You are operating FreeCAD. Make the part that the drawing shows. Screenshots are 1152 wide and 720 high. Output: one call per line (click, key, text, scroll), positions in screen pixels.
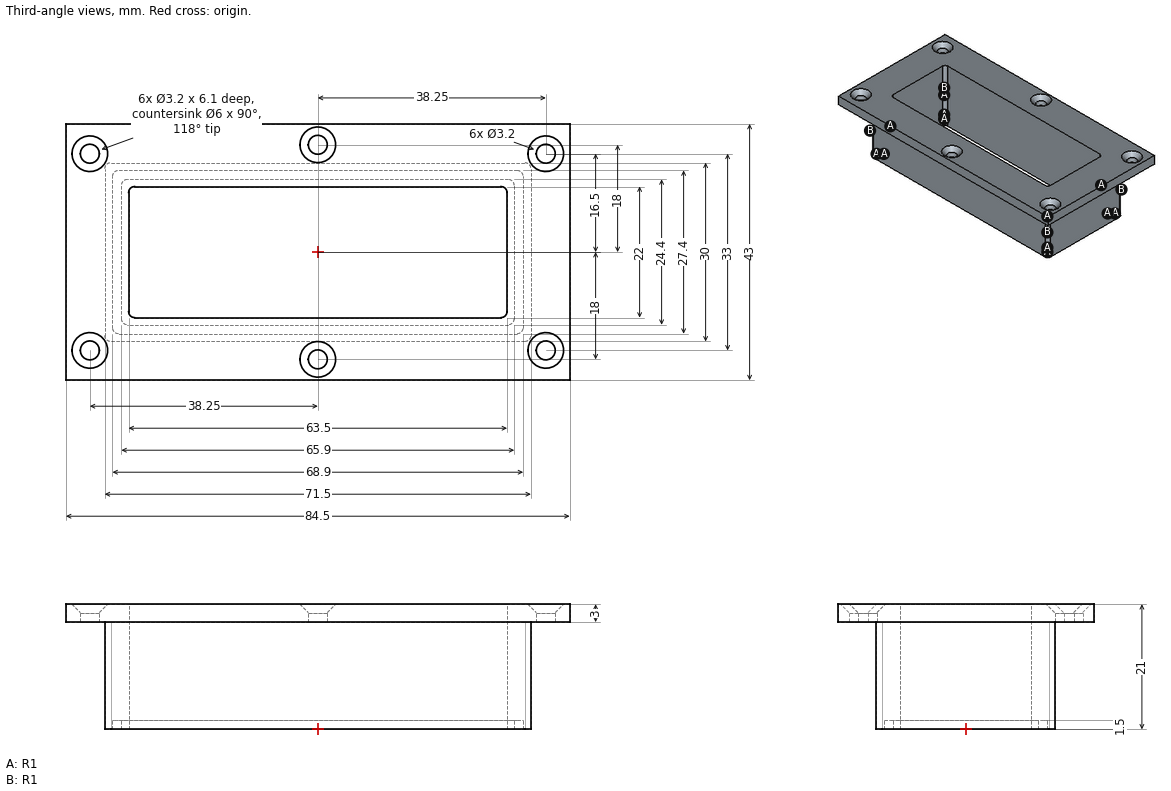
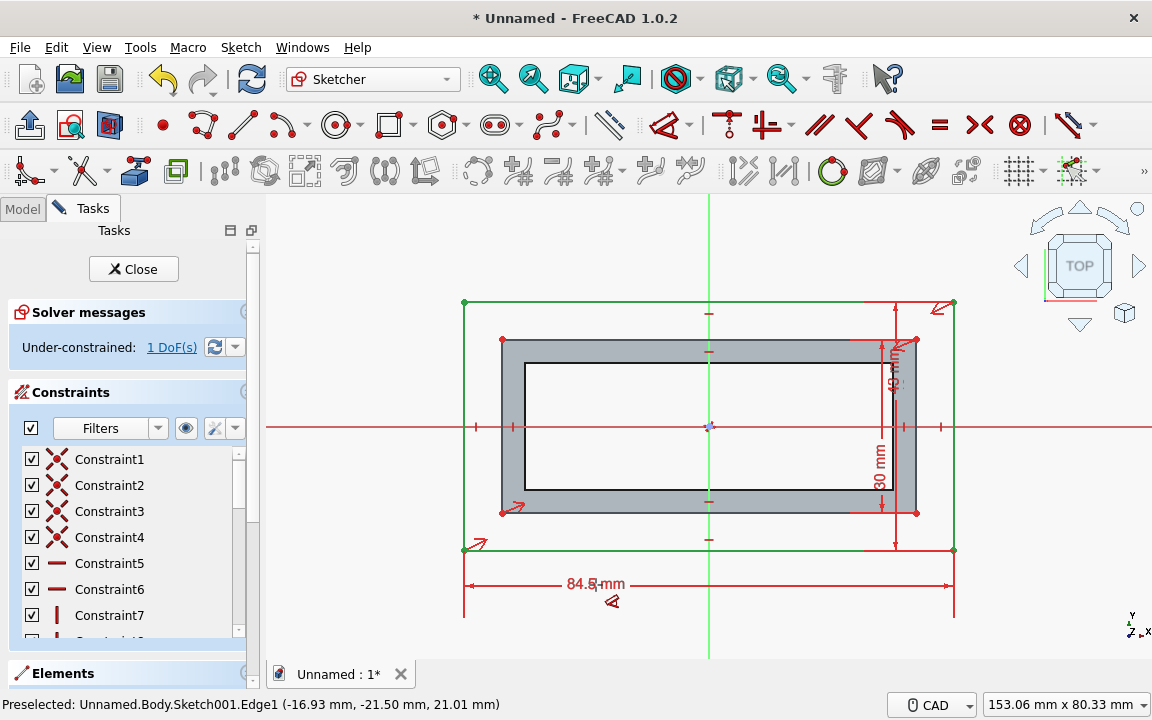
click(626, 513)
click(614, 479)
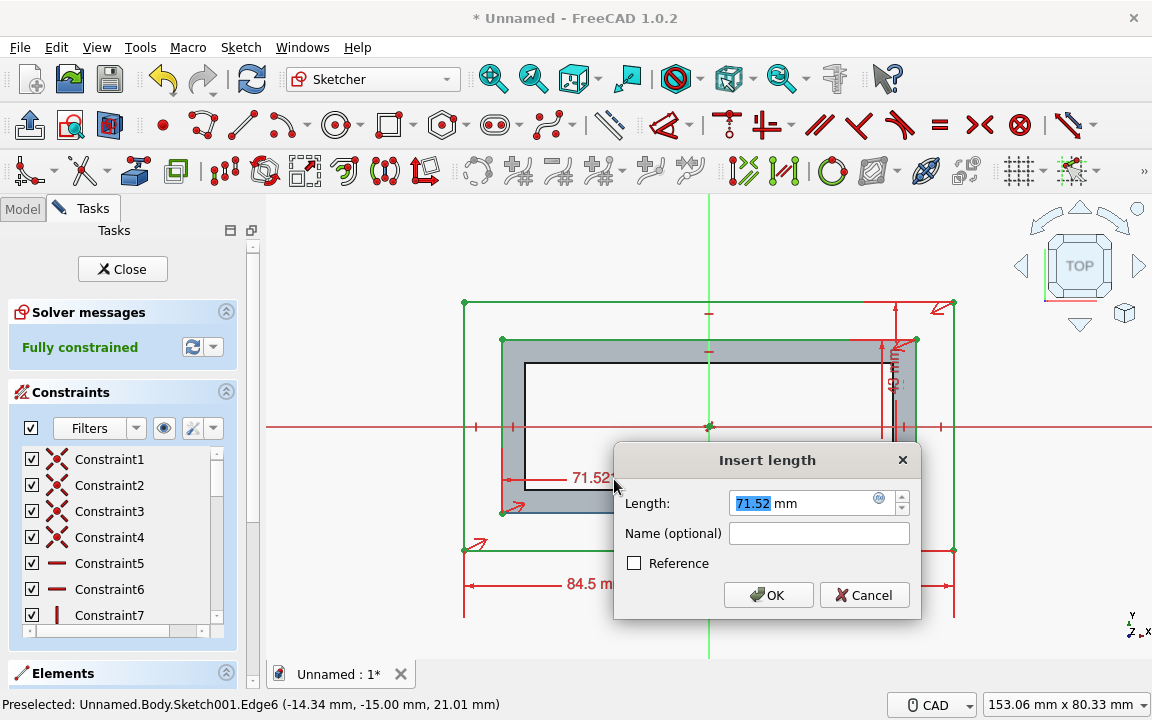
text(71.5)
key(Return)
key(Escape)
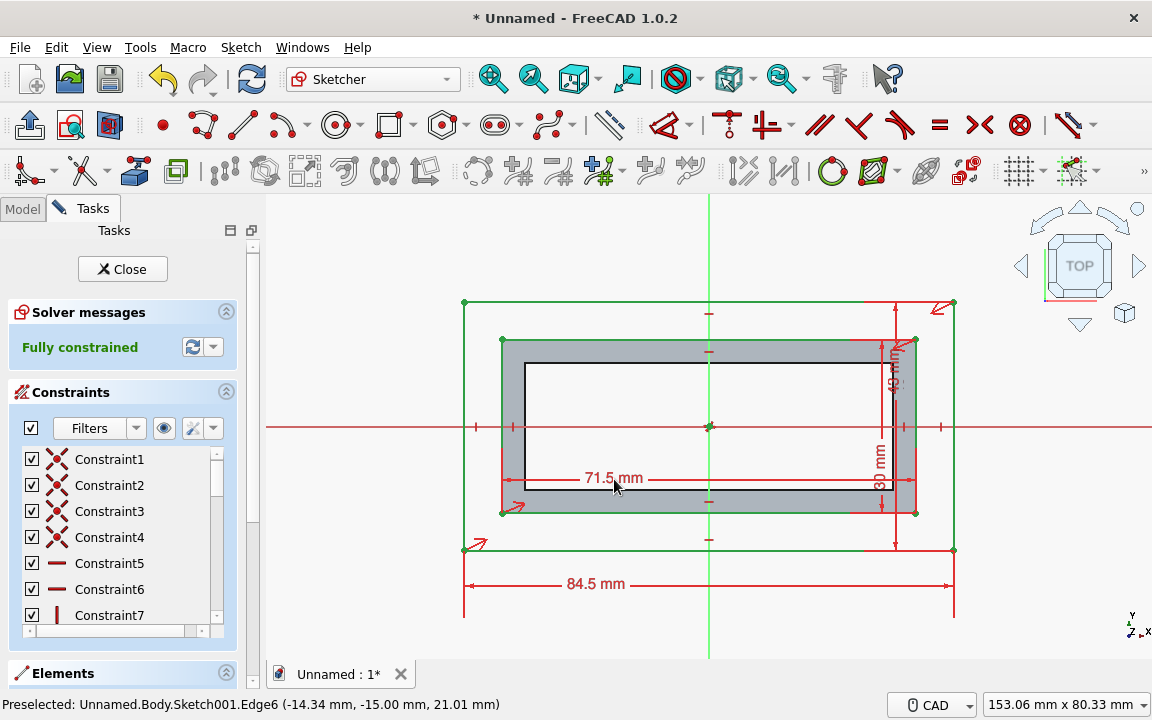
click(123, 269)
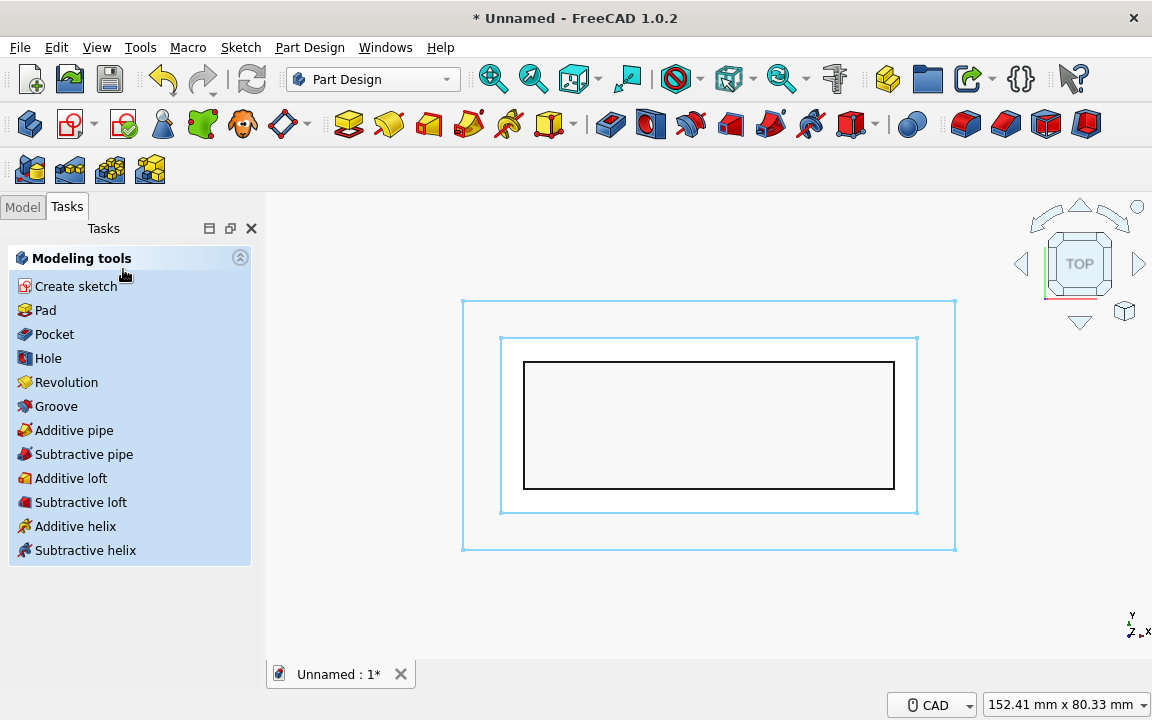
click(350, 124)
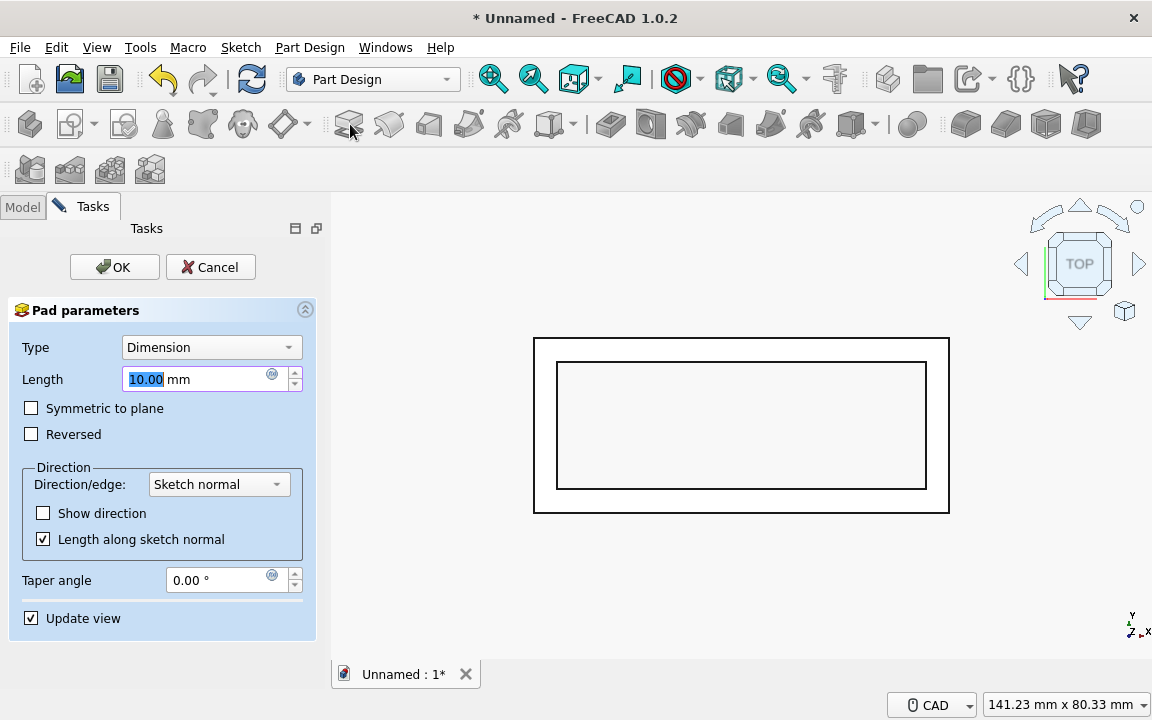
text(3)
key(Tab)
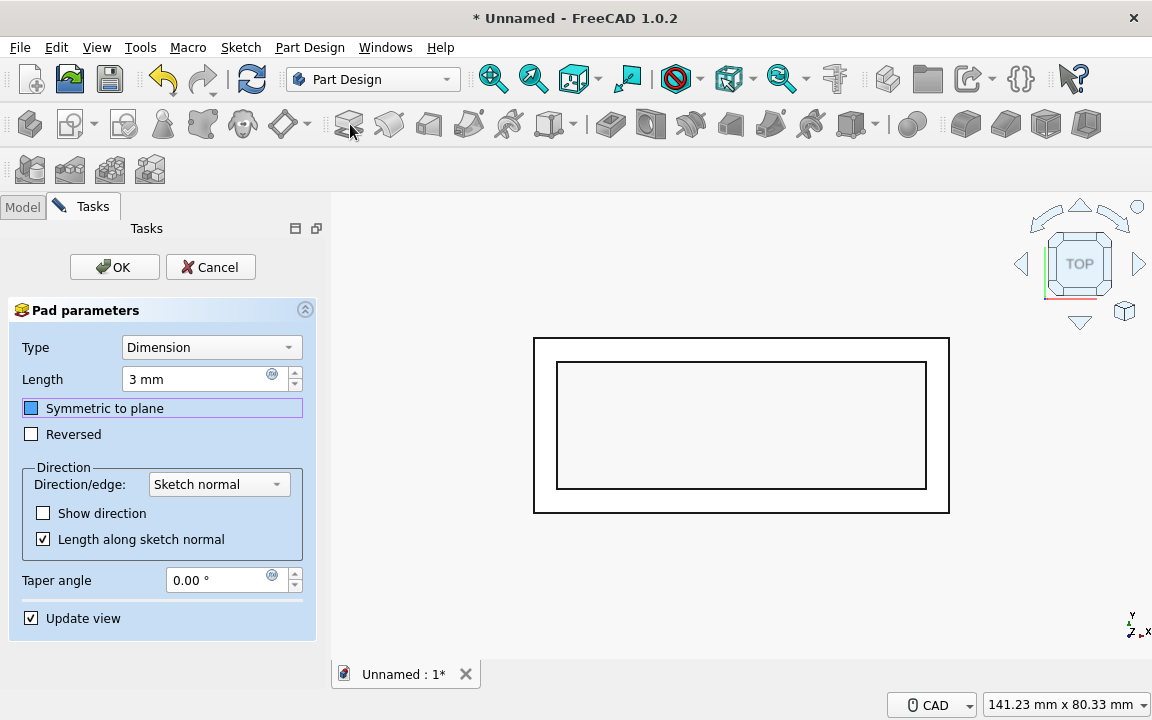
click(30, 434)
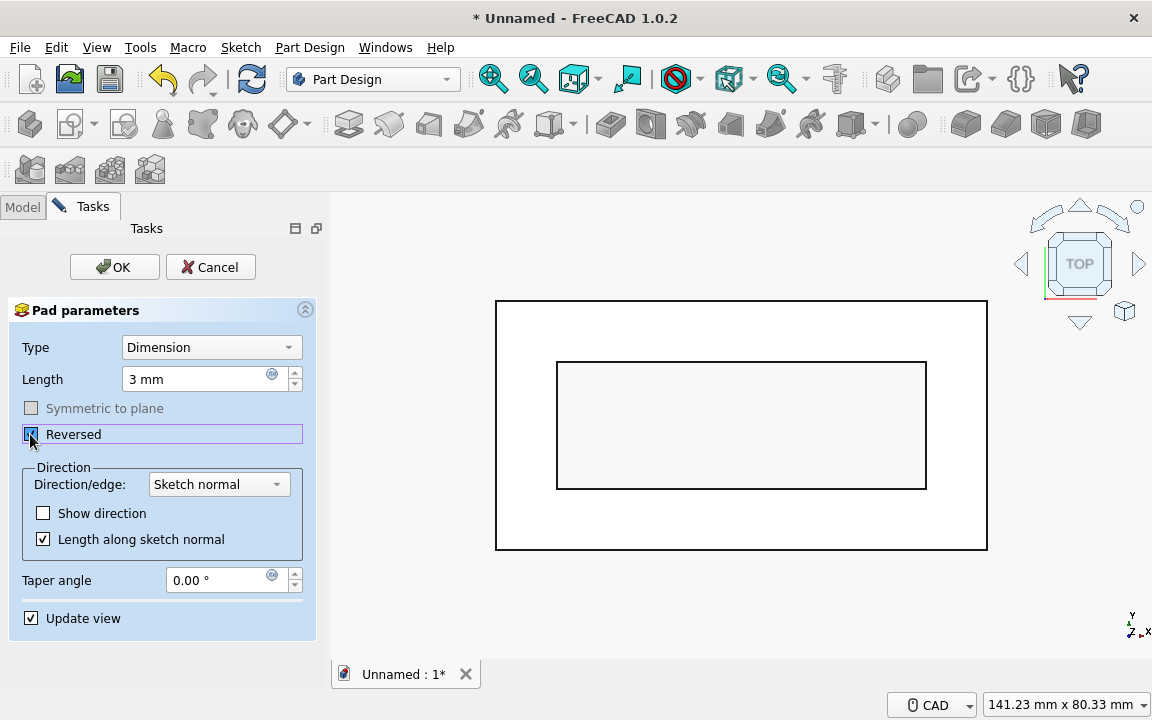
click(115, 267)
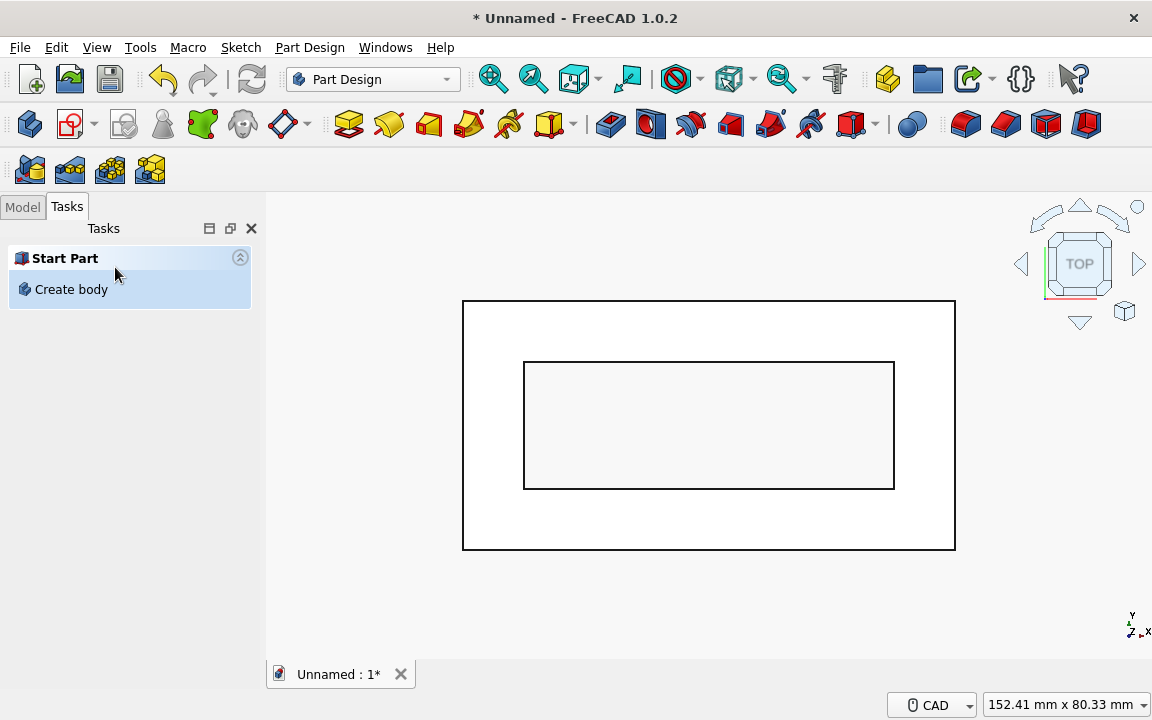
click(70, 124)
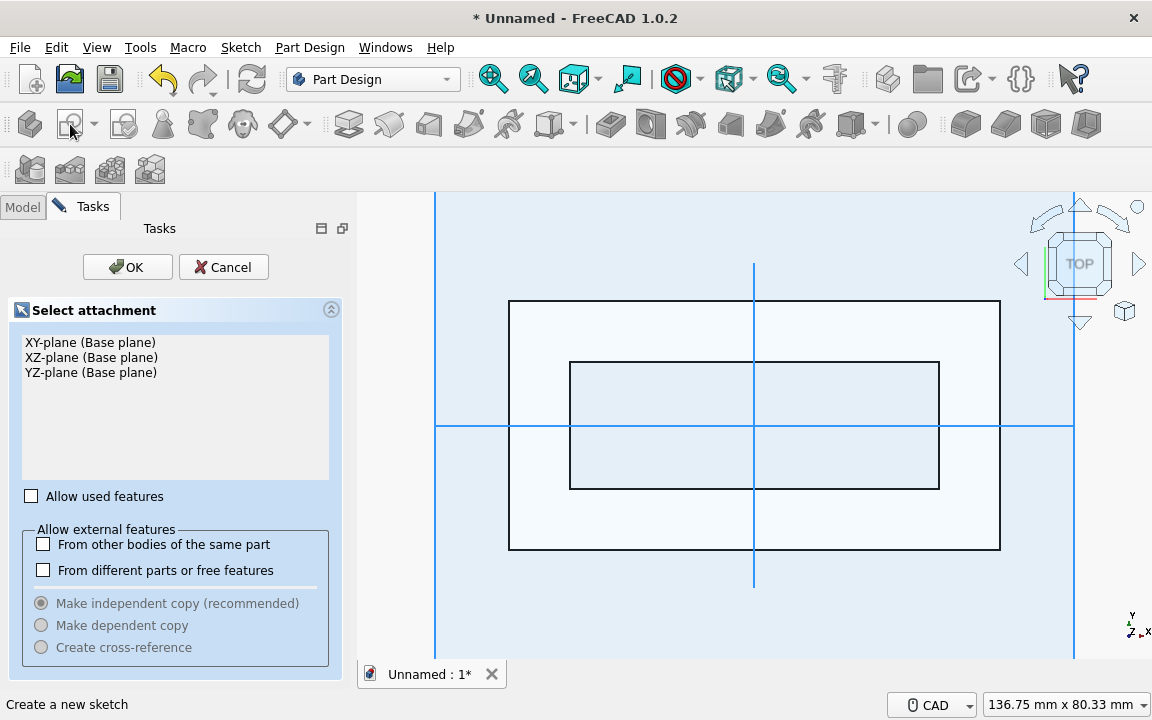
click(82, 342)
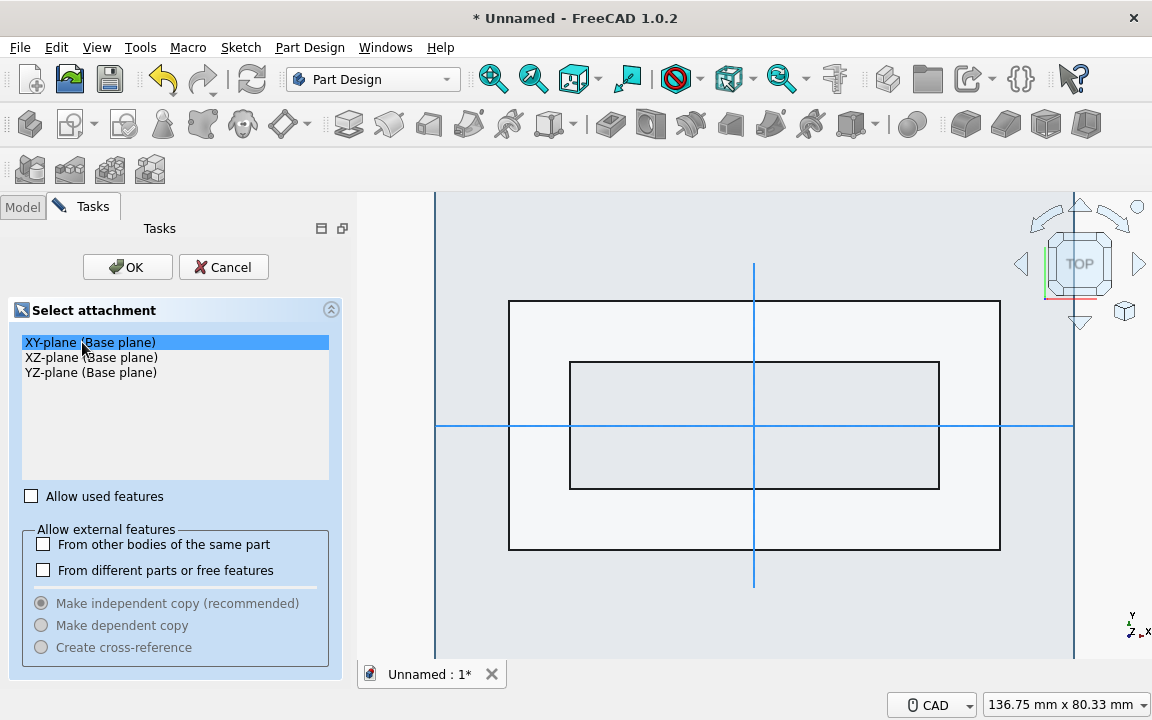
click(128, 267)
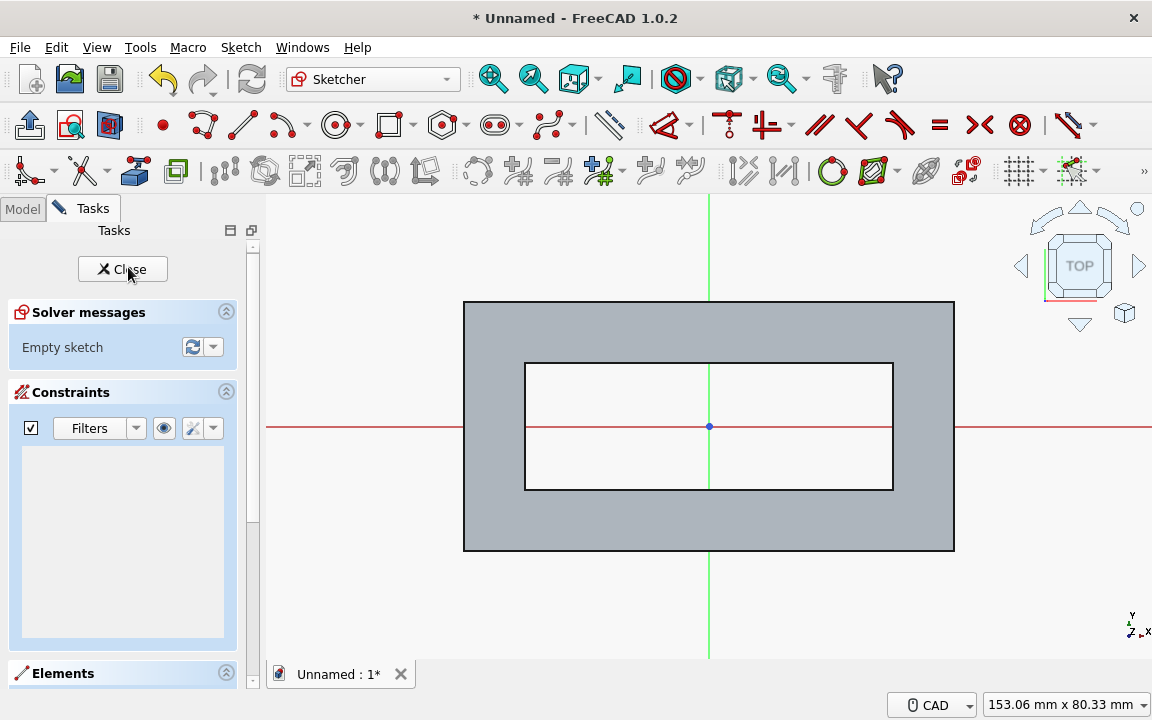
click(110, 126)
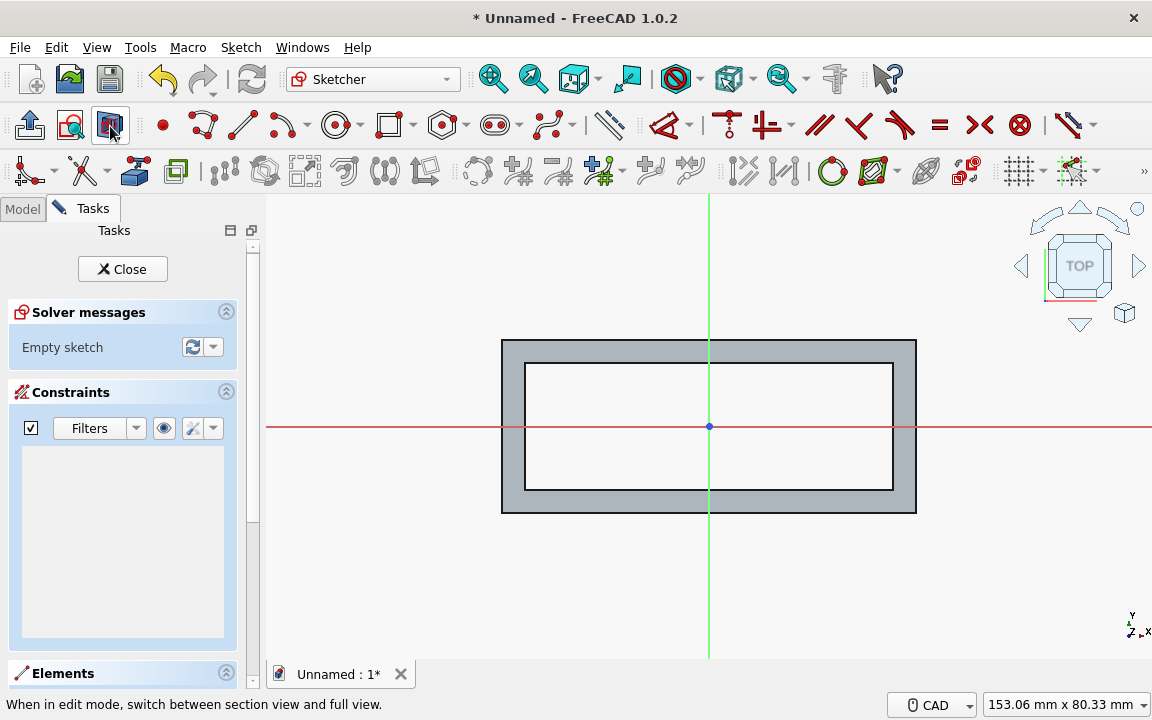
key(g)
key(v)